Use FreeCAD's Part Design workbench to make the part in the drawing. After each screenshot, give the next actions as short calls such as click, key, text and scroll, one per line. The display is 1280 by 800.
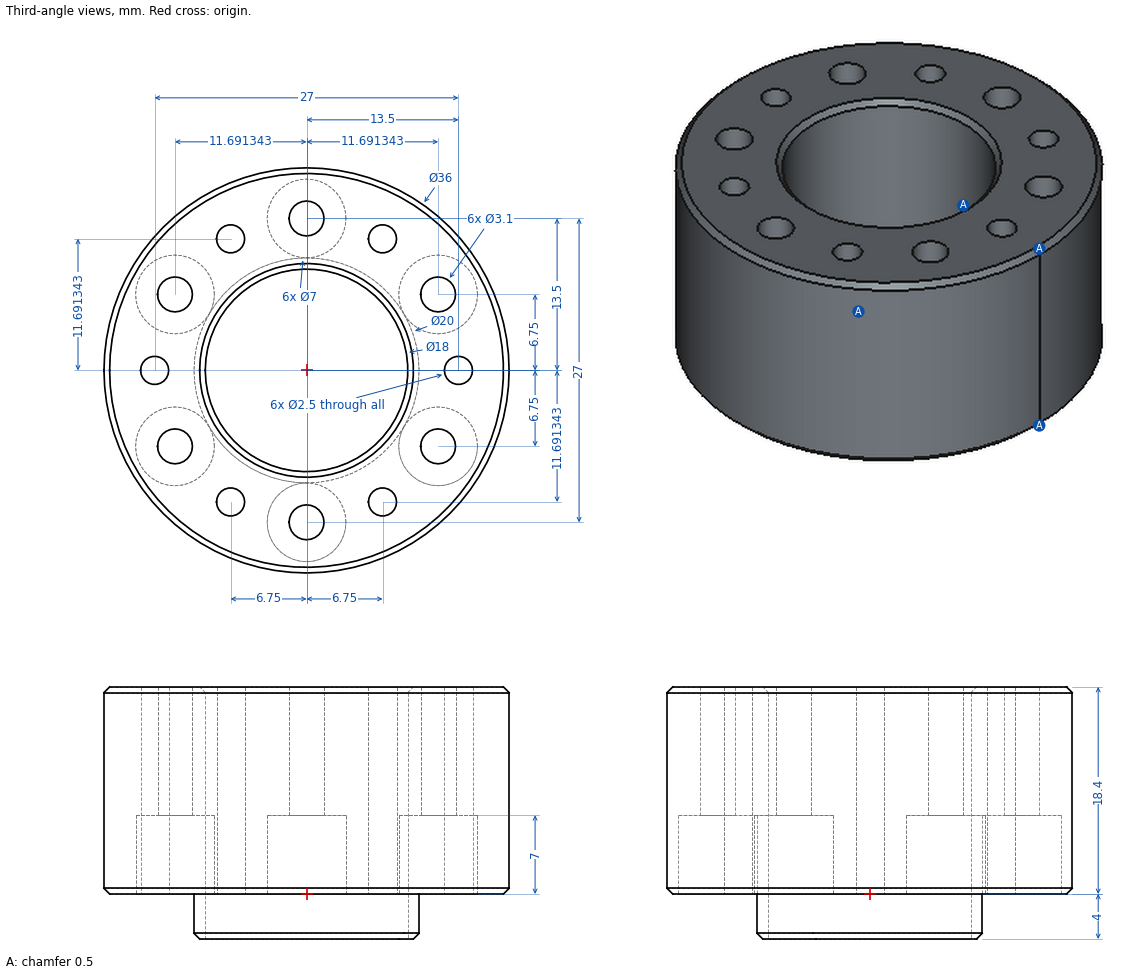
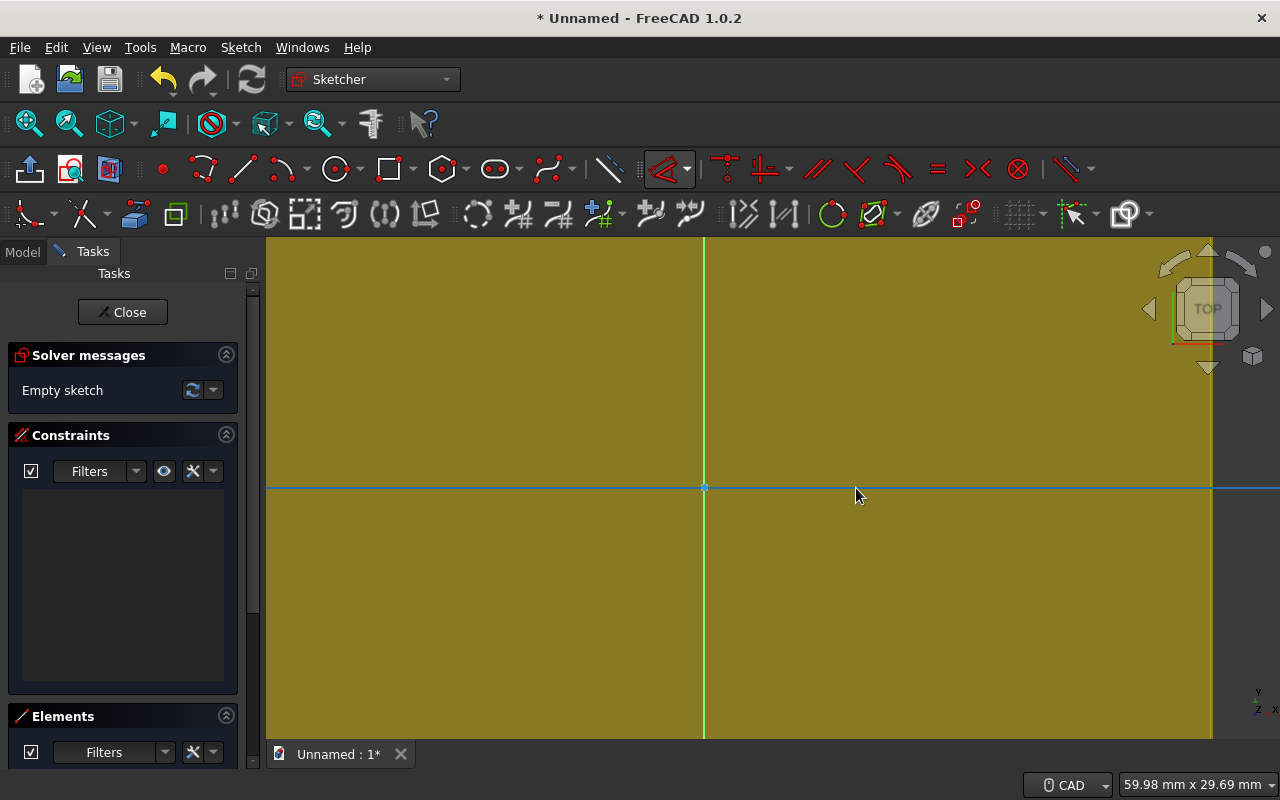
key(g)
key(c)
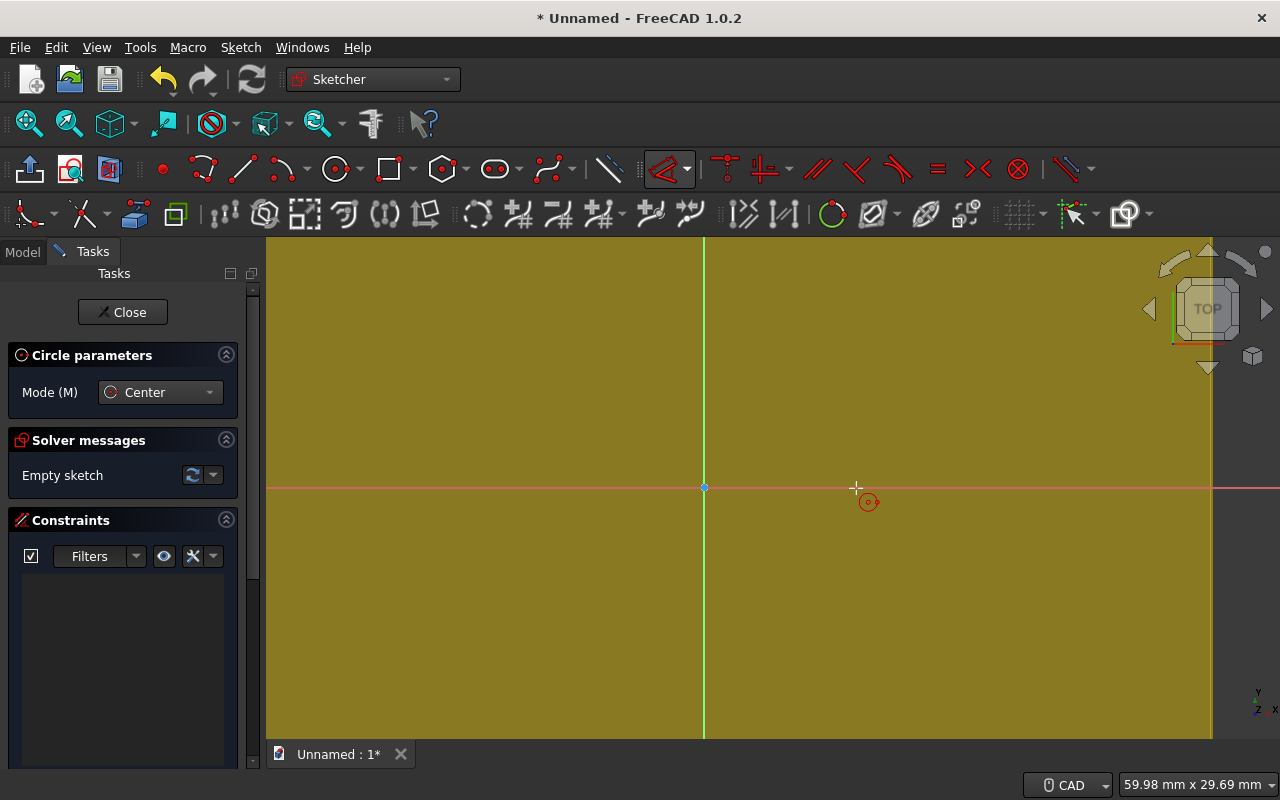
click(704, 488)
click(824, 368)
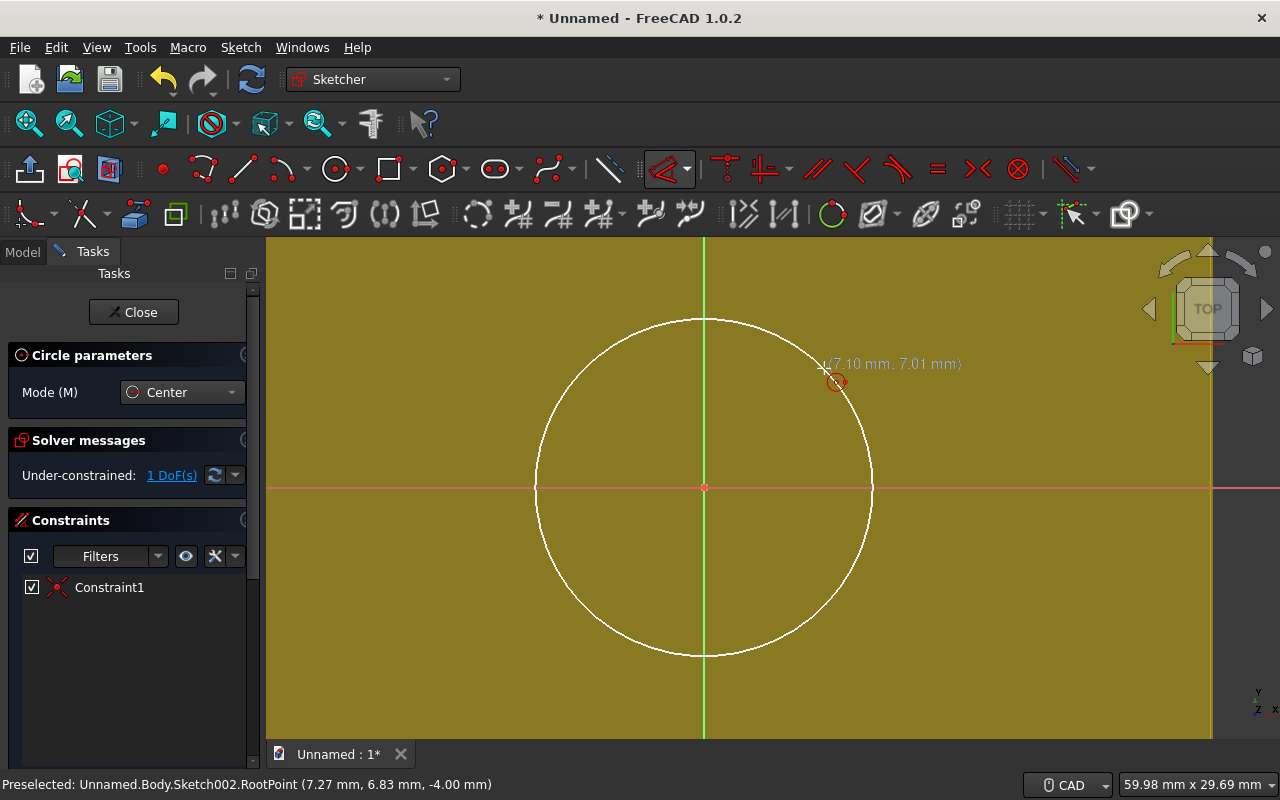
click(704, 488)
click(812, 380)
key(Escape)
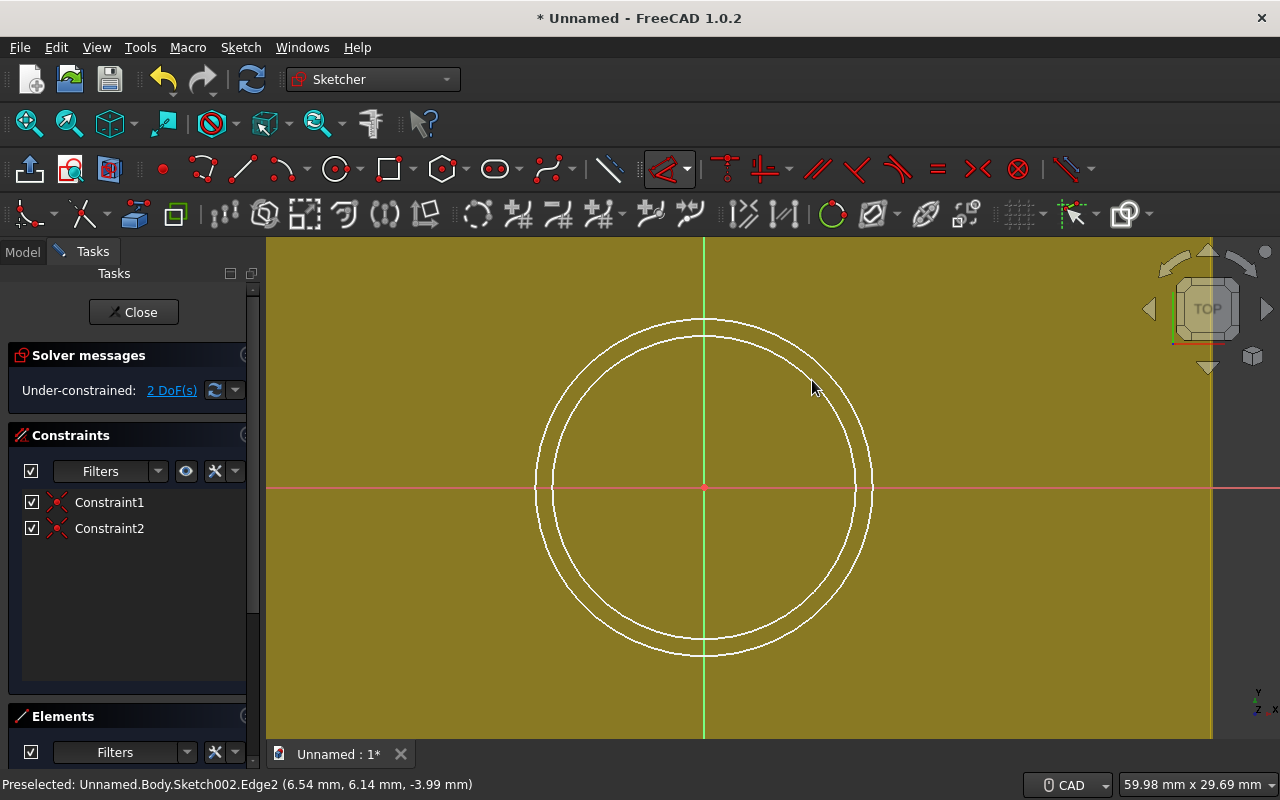
click(823, 368)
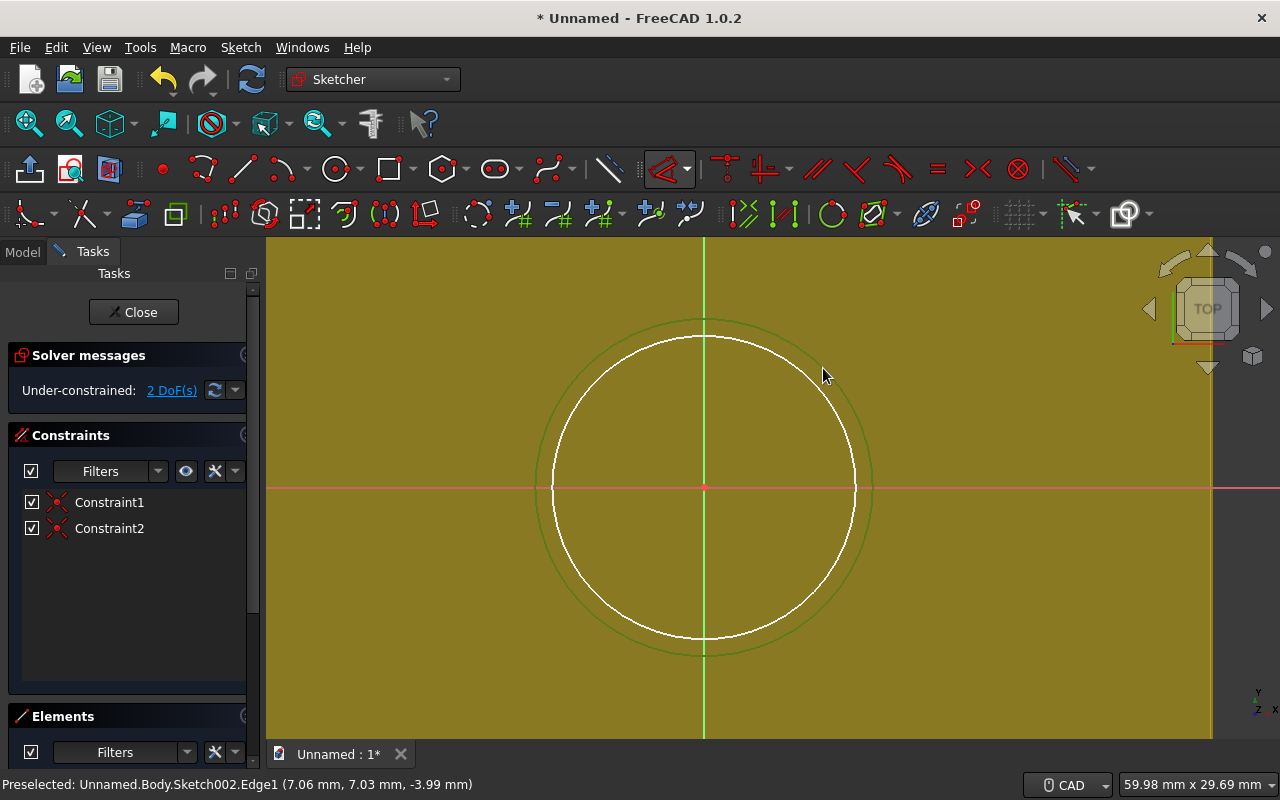
key(k)
key(o)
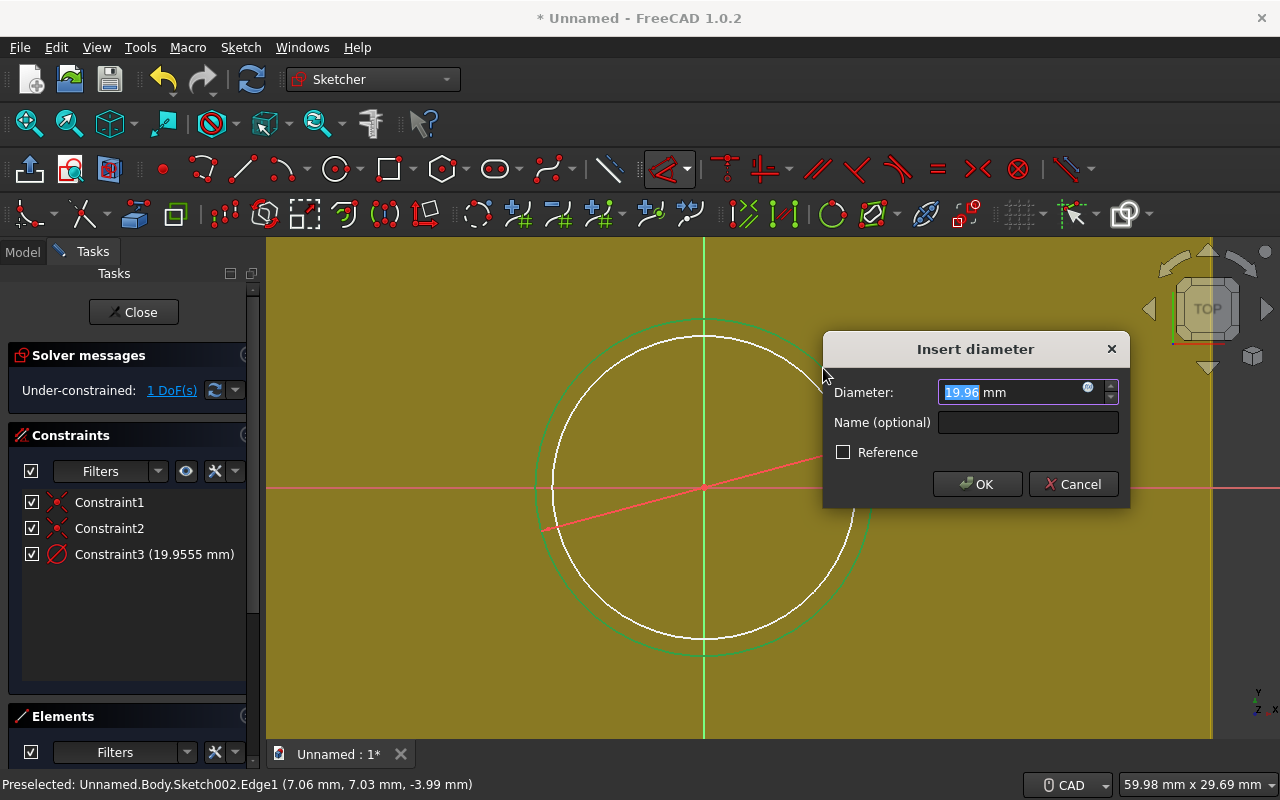
text(20)
key(Return)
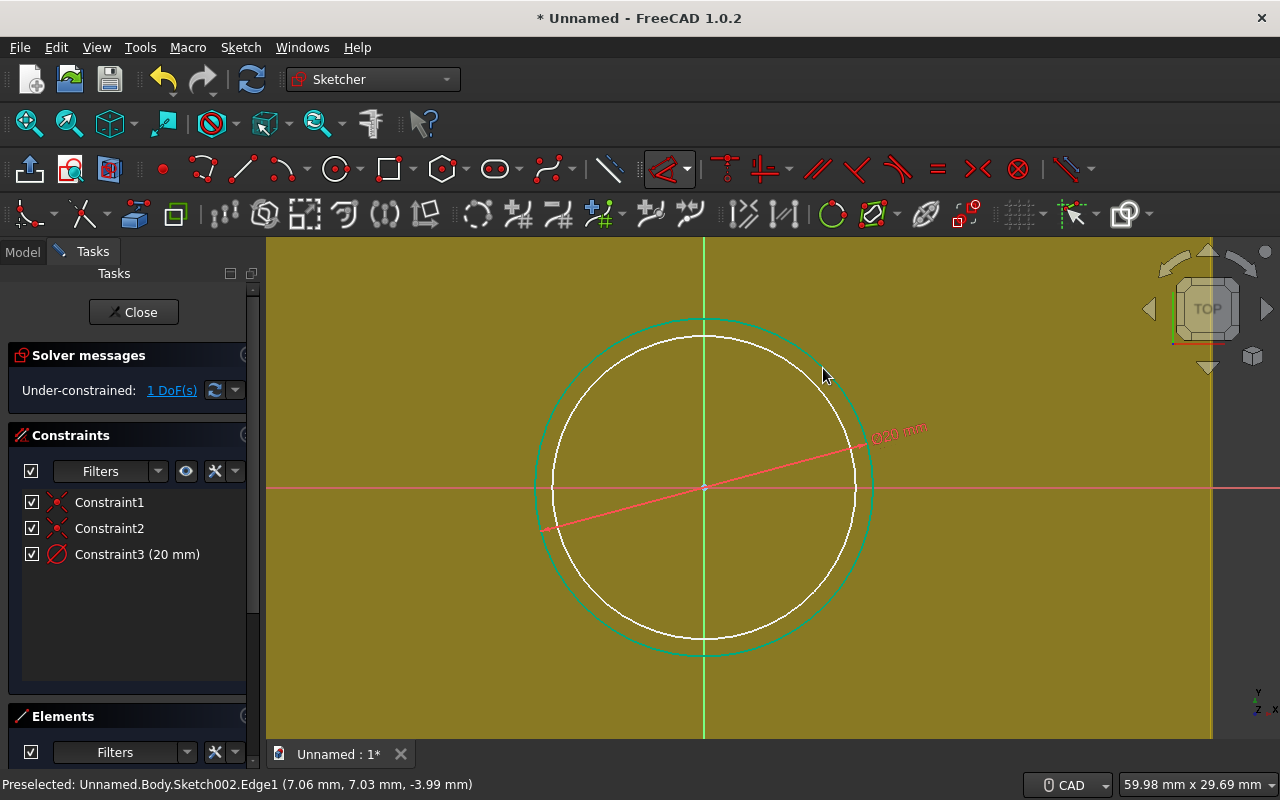
click(811, 380)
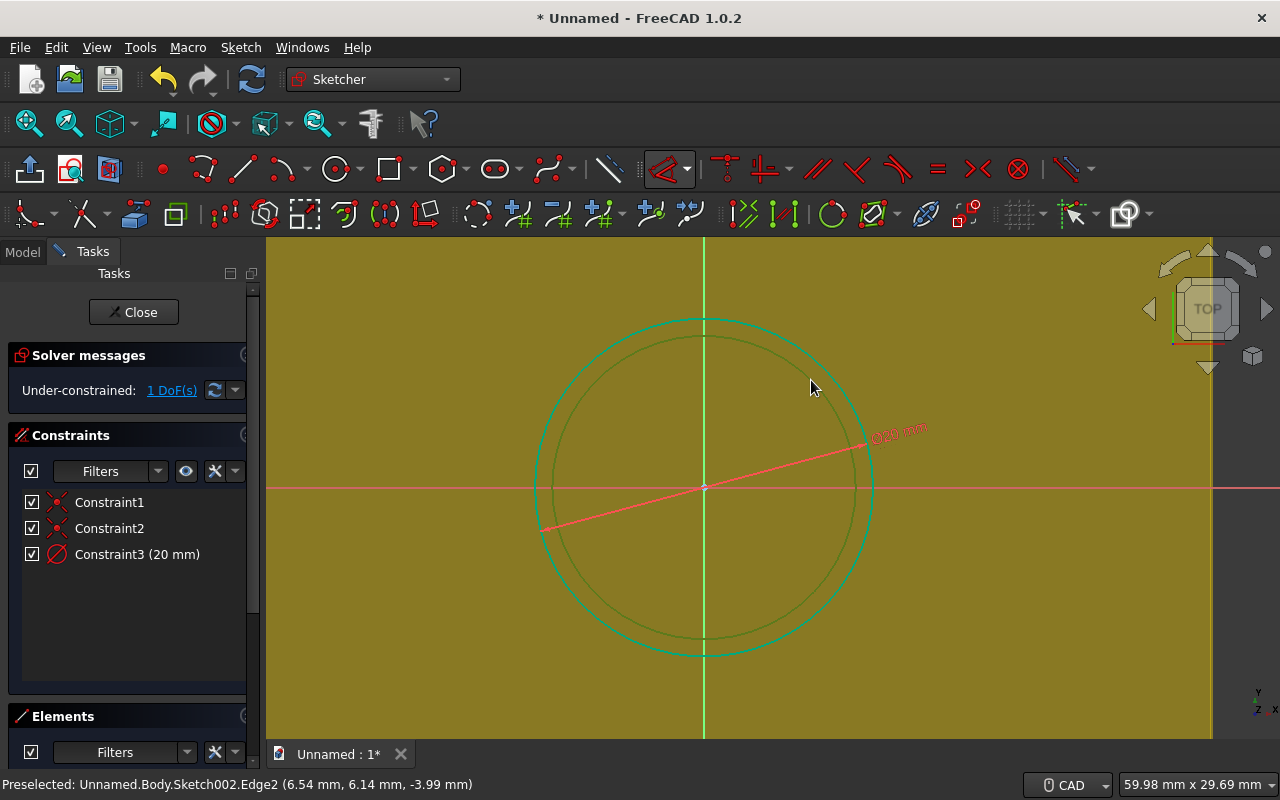
click(690, 170)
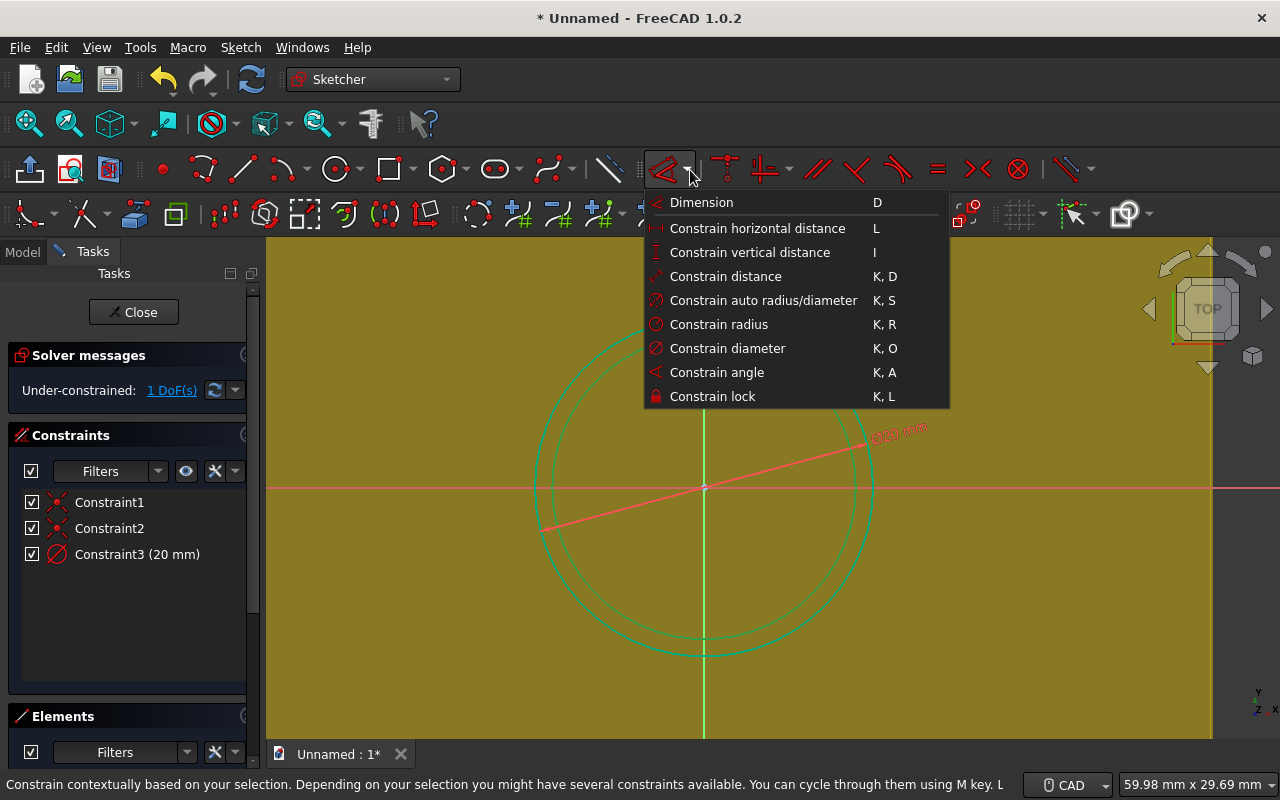
click(797, 348)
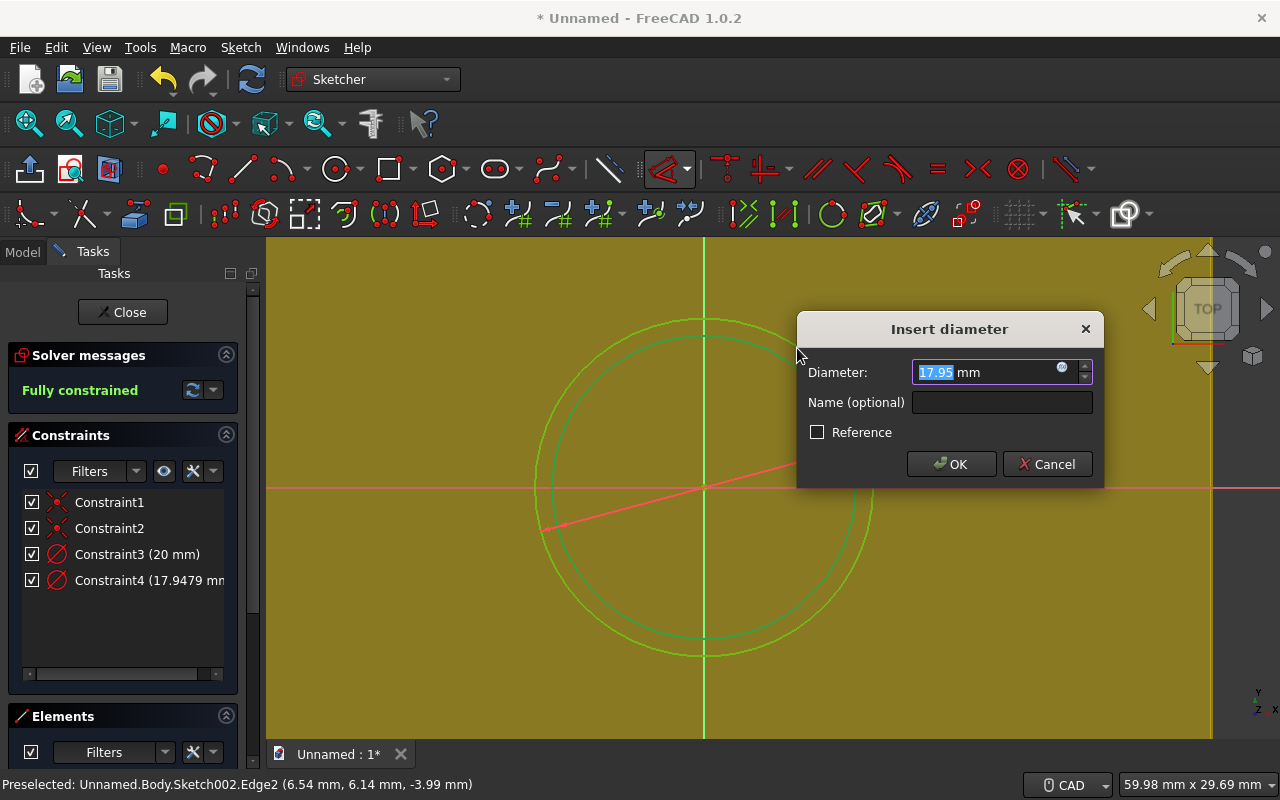
text(18)
key(Return)